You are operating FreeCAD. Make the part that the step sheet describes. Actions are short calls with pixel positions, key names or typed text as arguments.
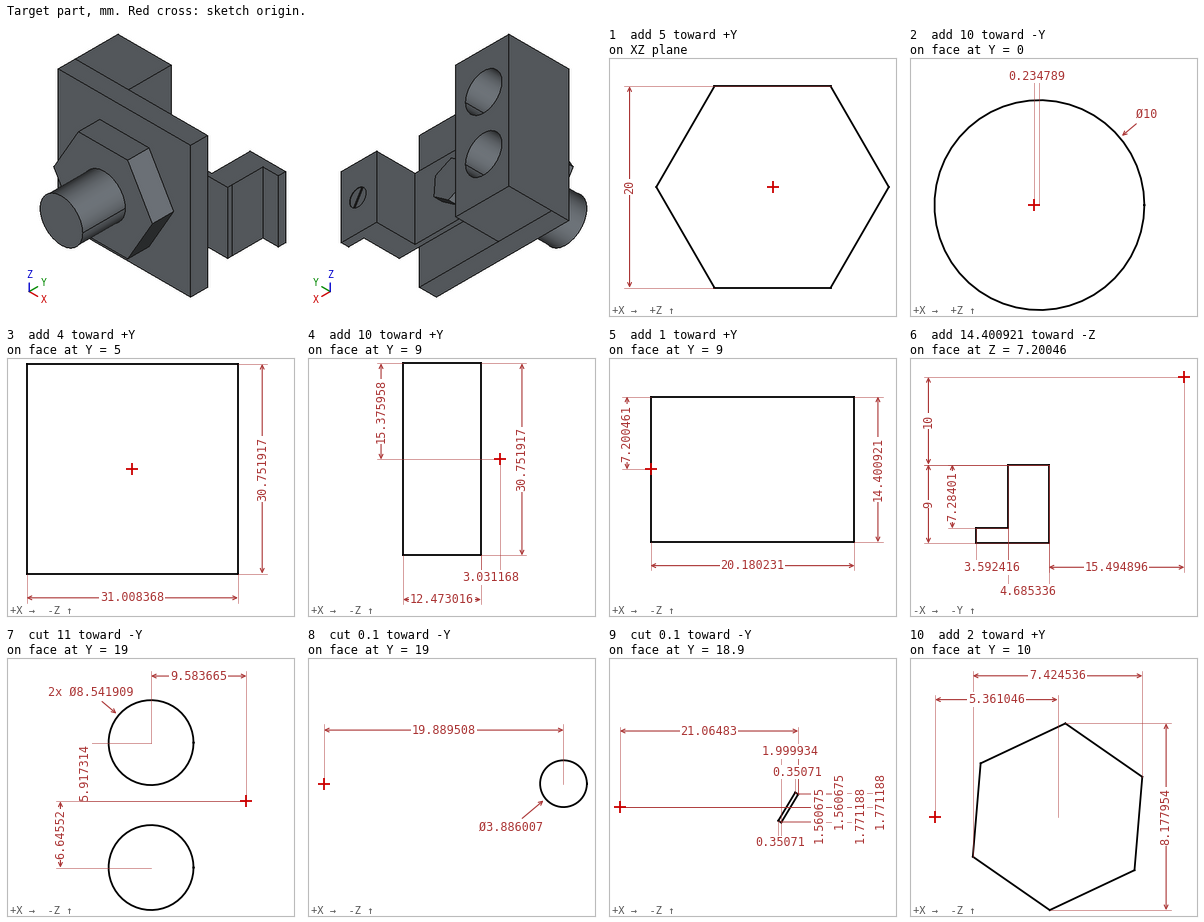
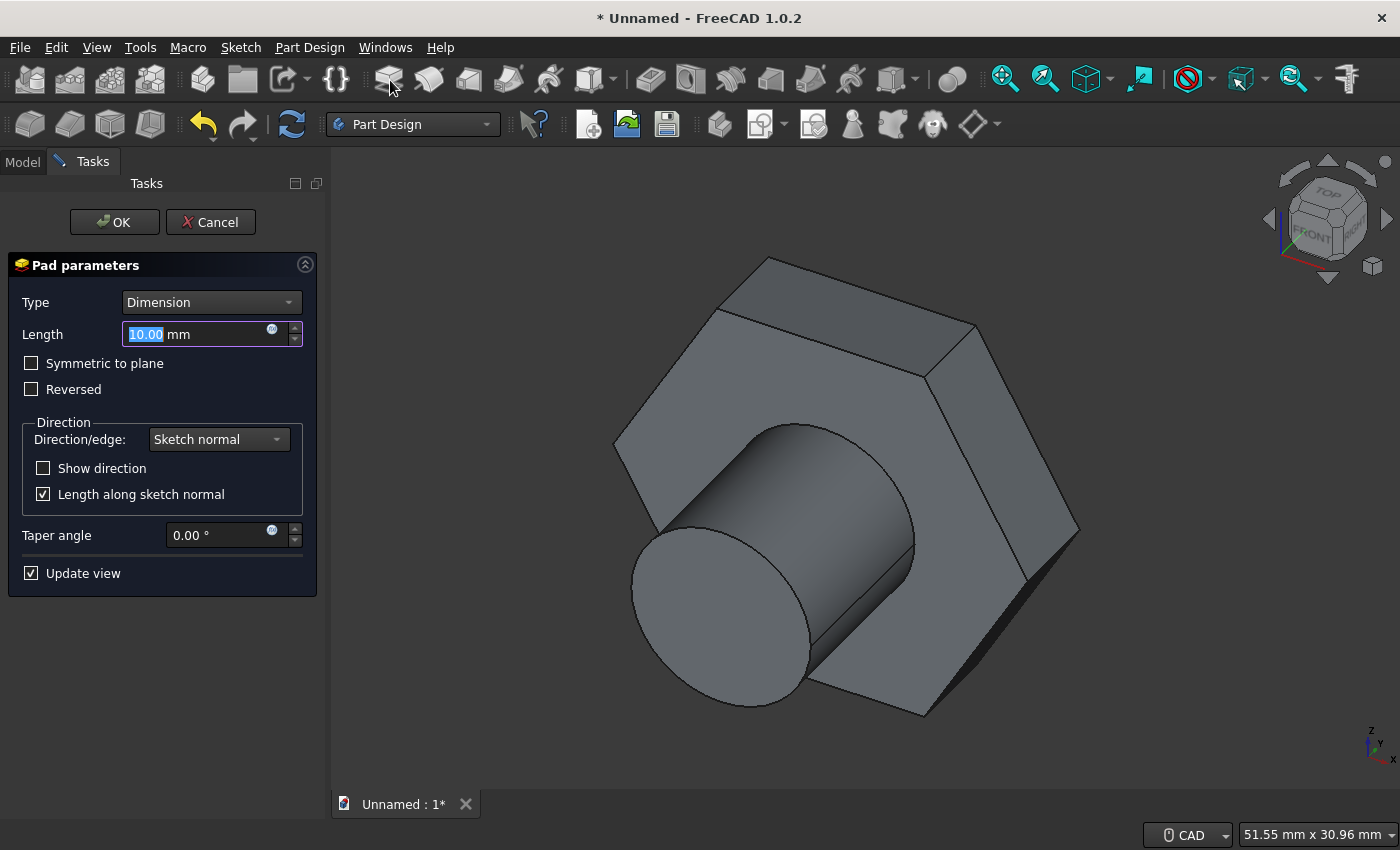
text(10)
key(Tab)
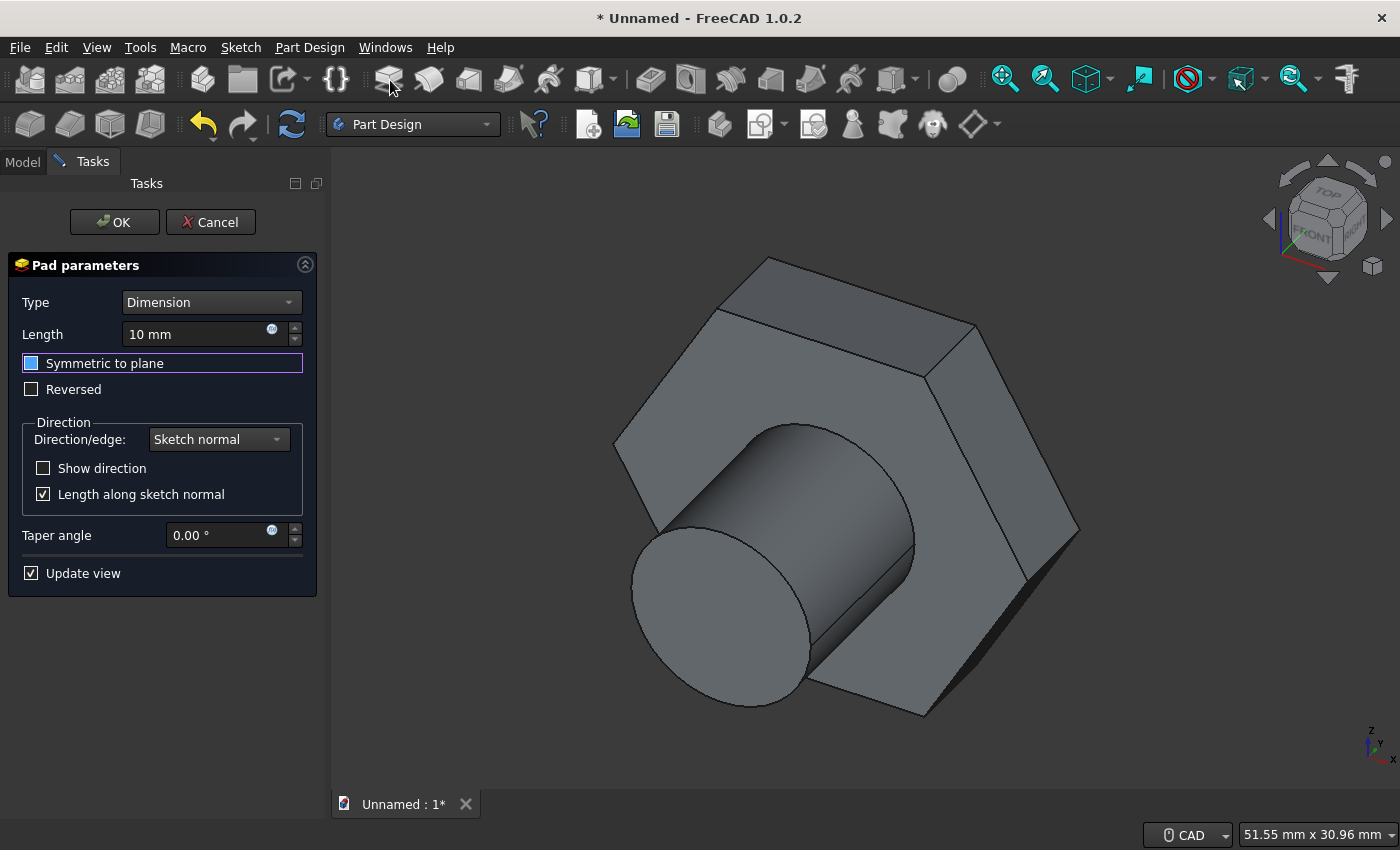
click(115, 222)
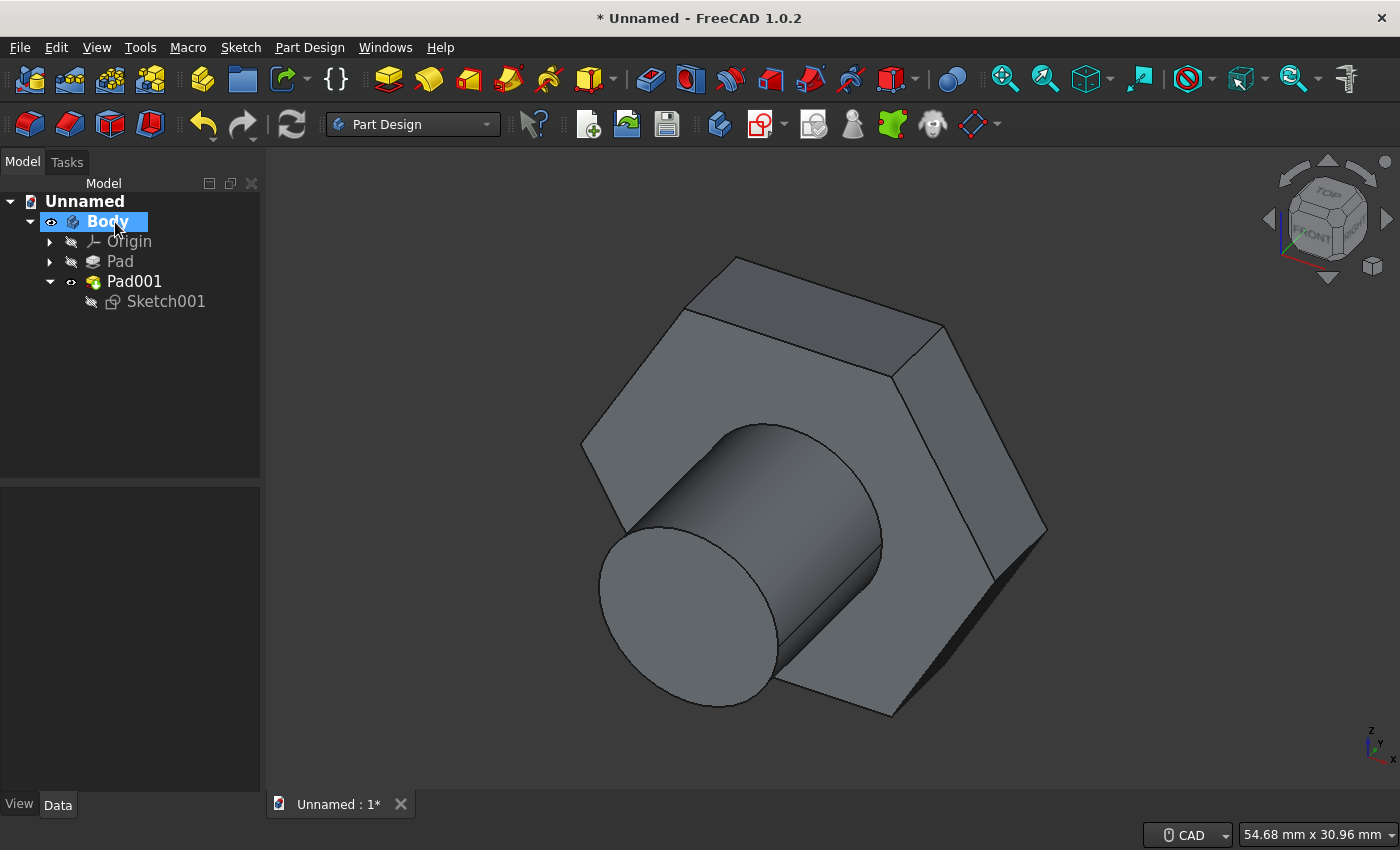
click(1006, 80)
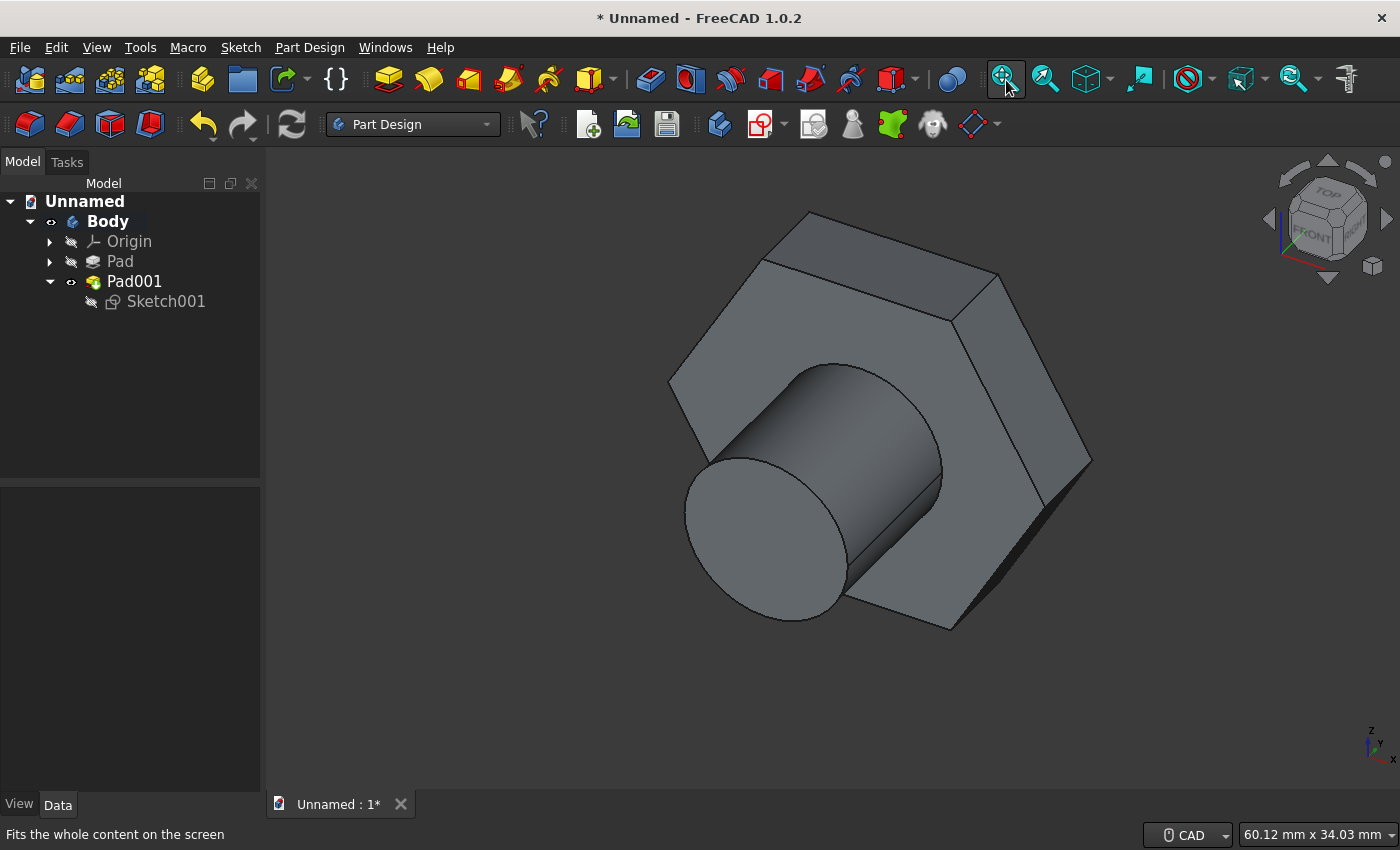
key(4)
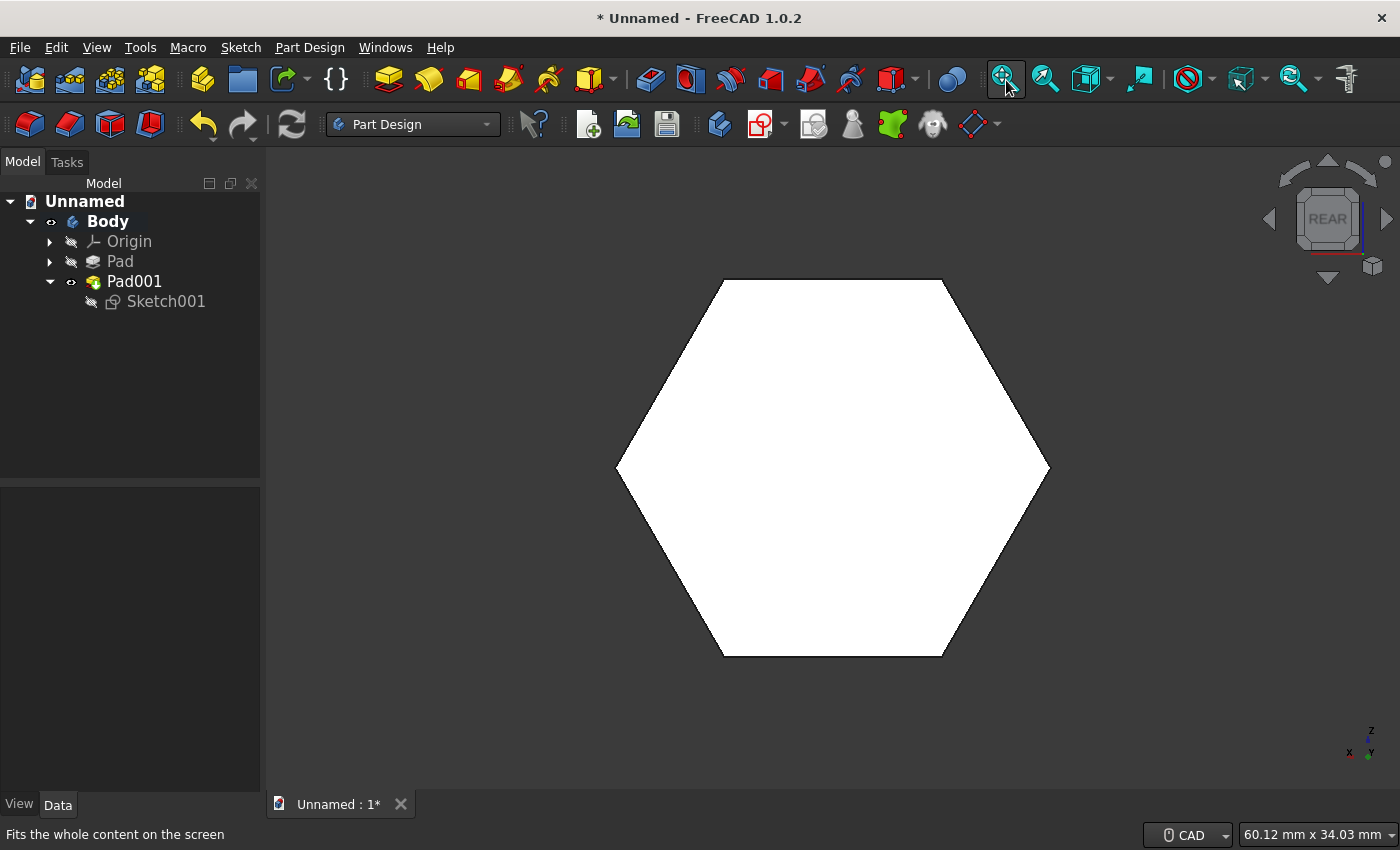
click(833, 467)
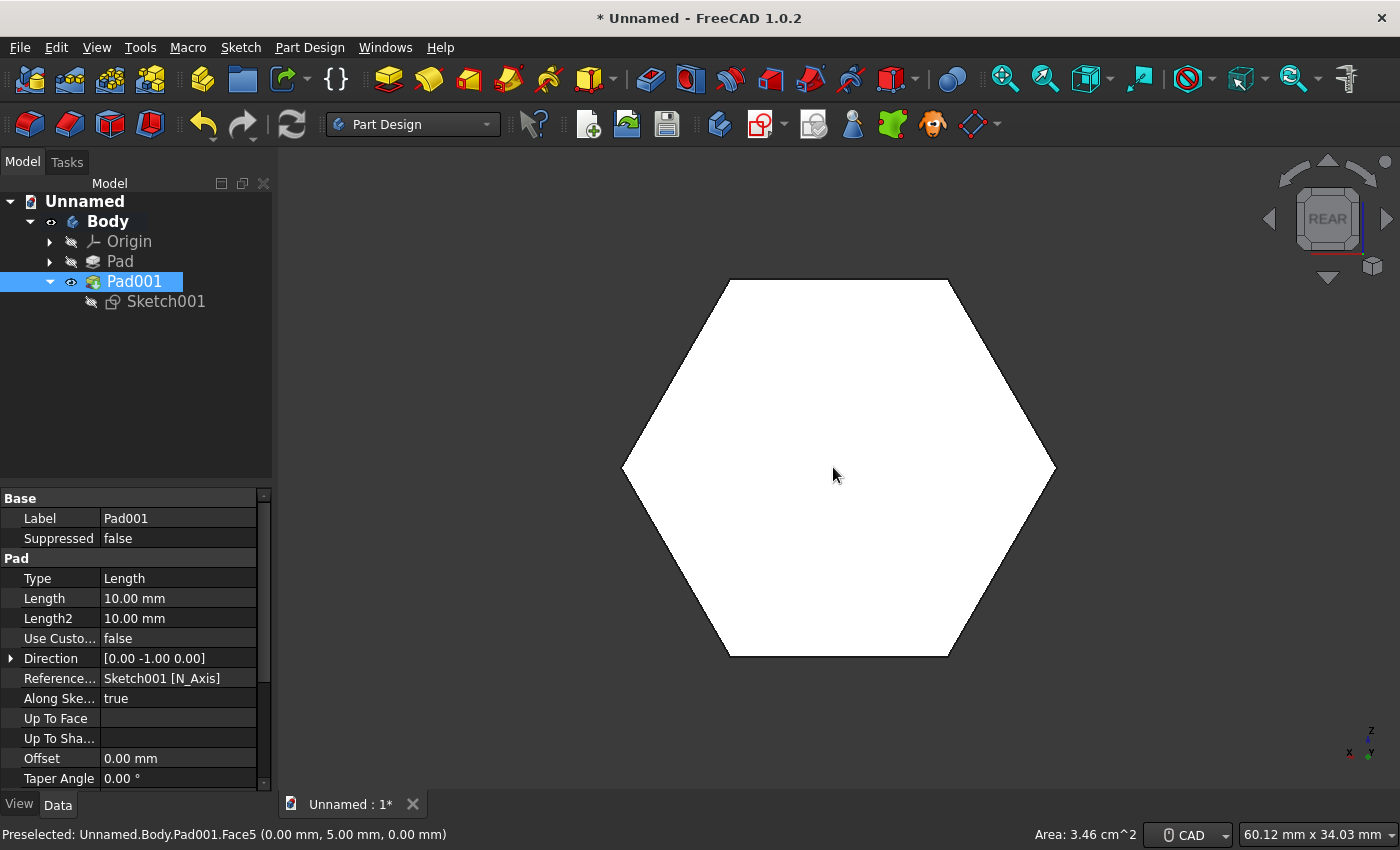
click(760, 124)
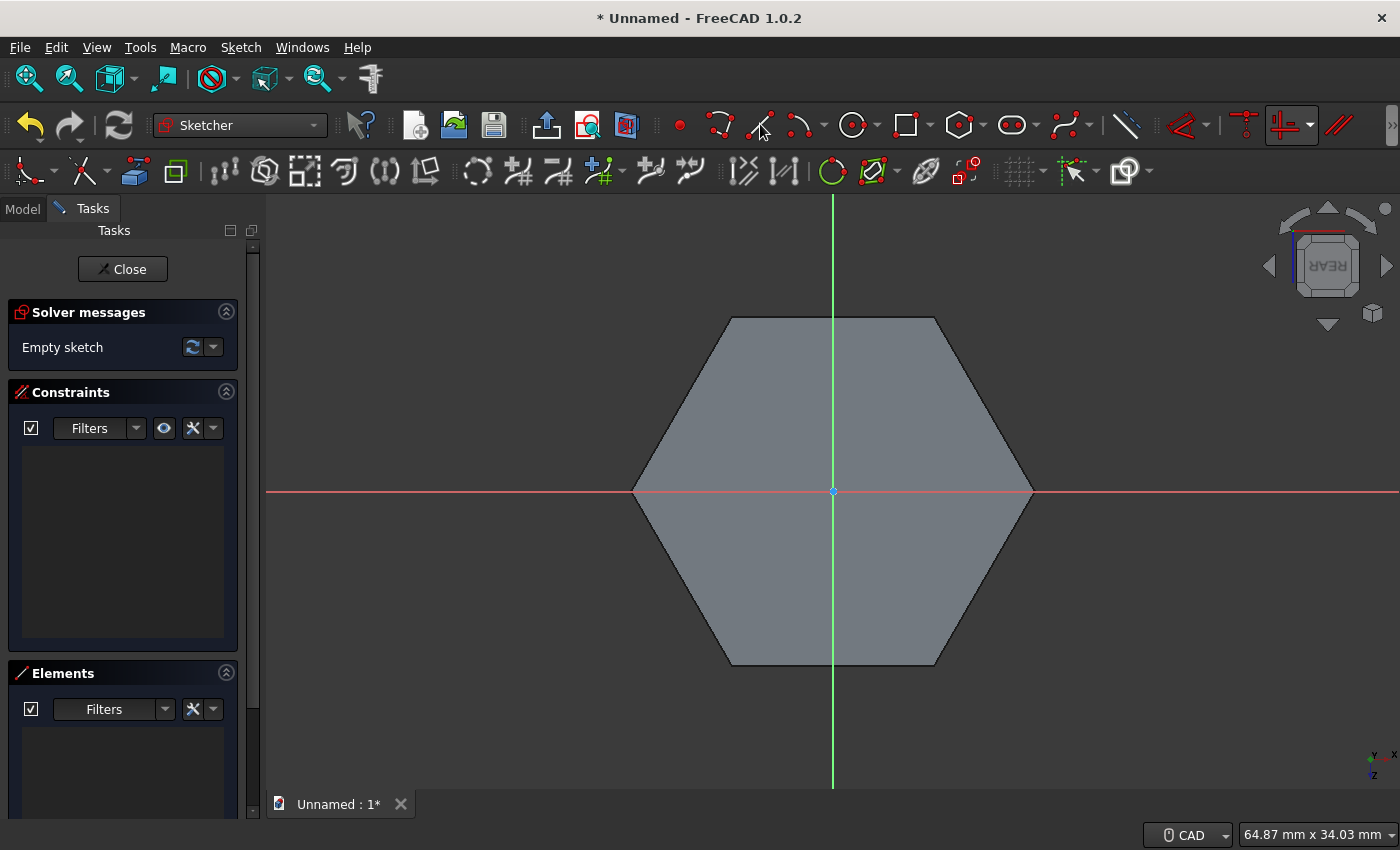
scroll(625, 491, down, 2)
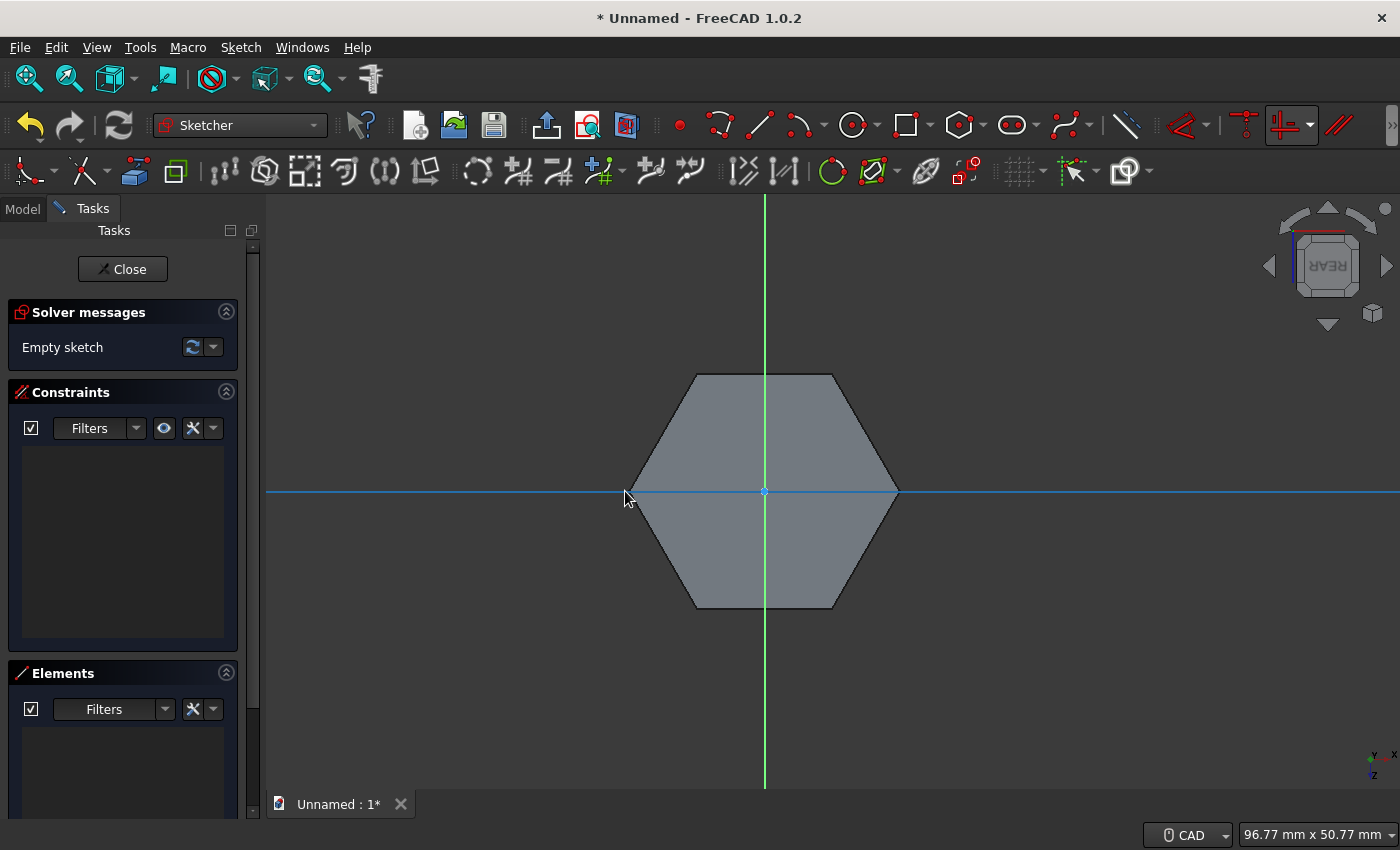
key(g)
key(v)